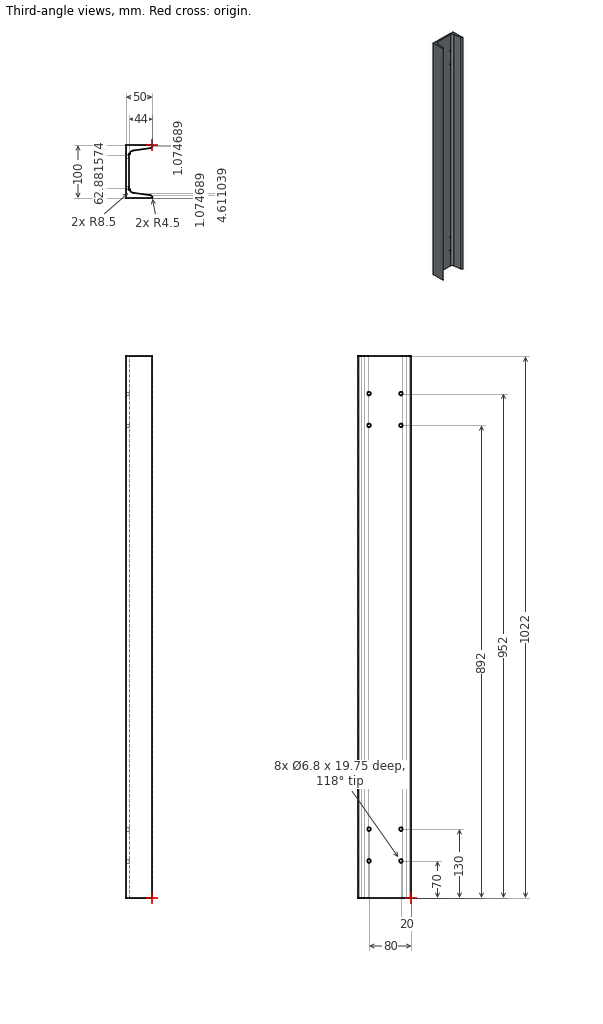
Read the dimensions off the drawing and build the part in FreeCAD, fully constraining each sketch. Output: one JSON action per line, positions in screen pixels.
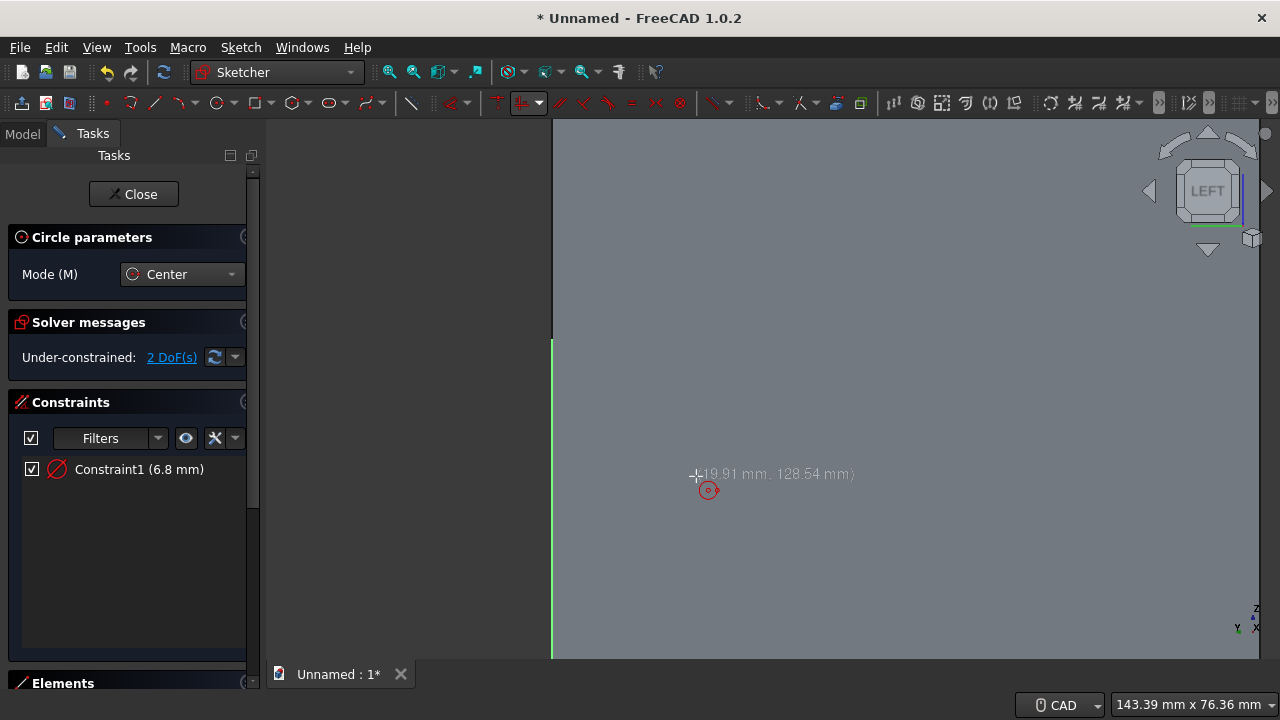
{"action": "scroll", "coordinate": [697, 514], "scroll_direction": "down", "scroll_amount": 15}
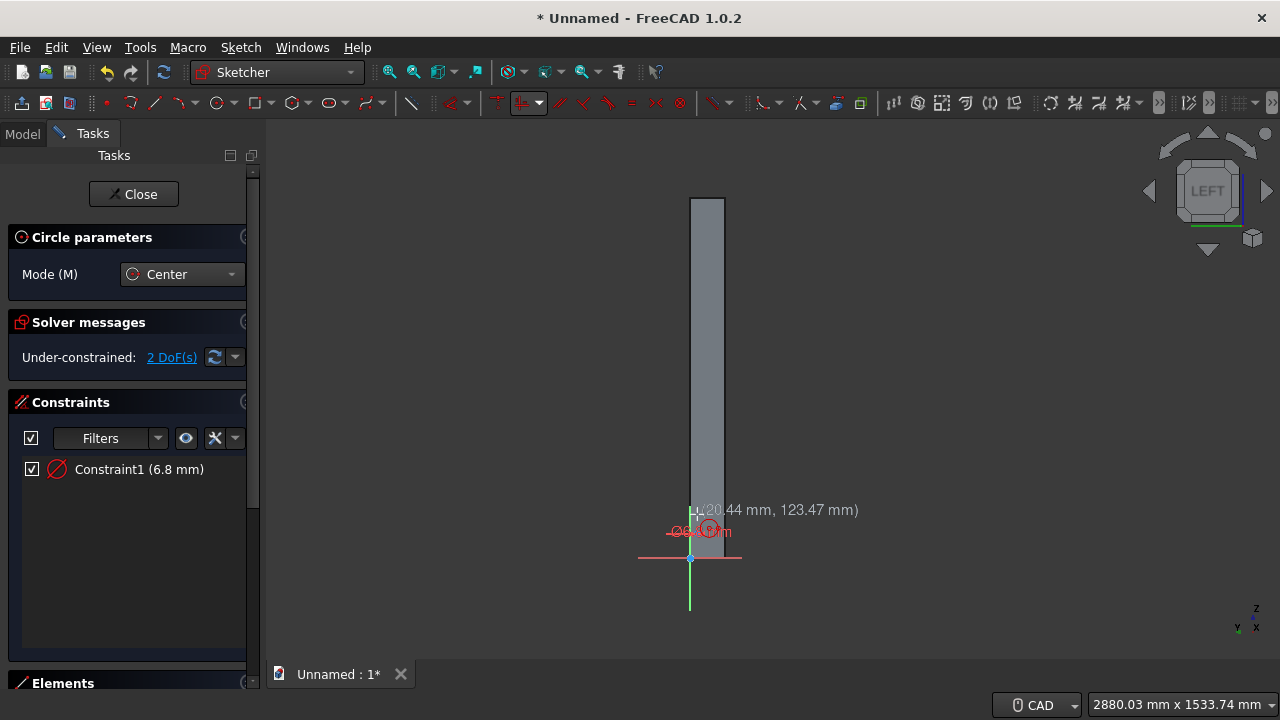
{"action": "scroll", "coordinate": [697, 512], "scroll_direction": "up", "scroll_amount": 5}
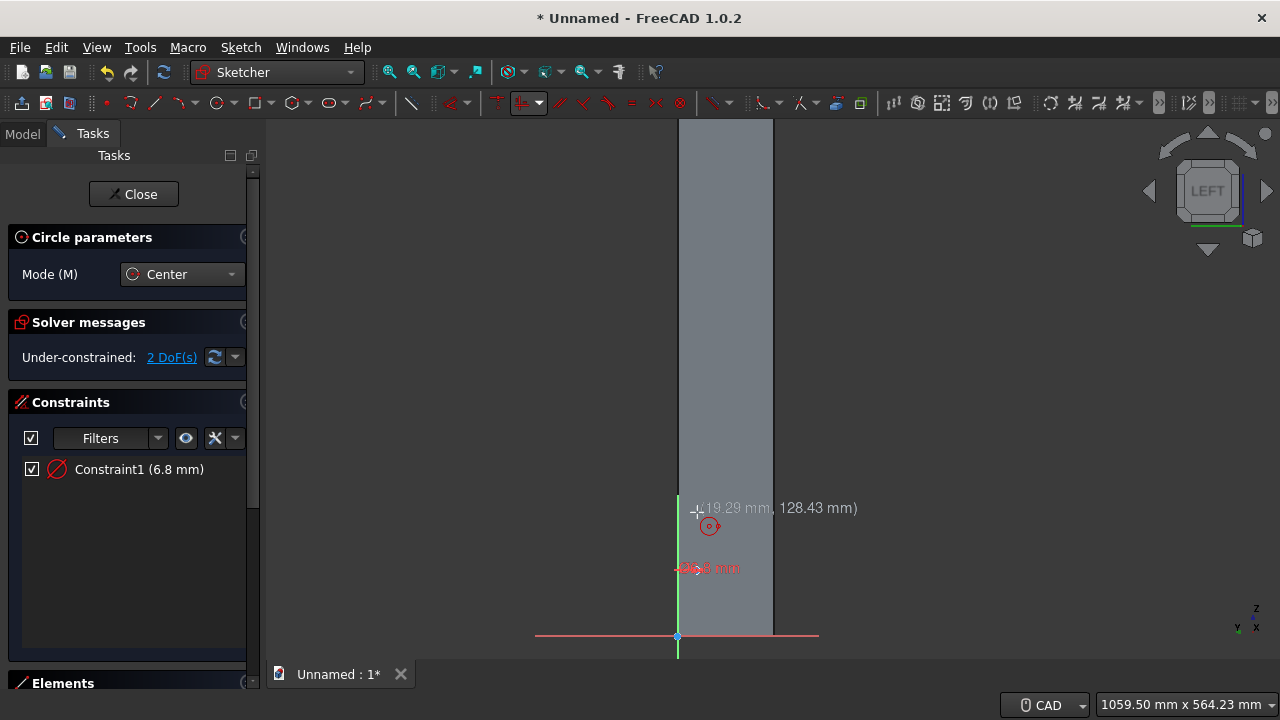
{"action": "left_click", "coordinate": [697, 512]}
{"action": "mouse_move", "coordinate": [699, 510]}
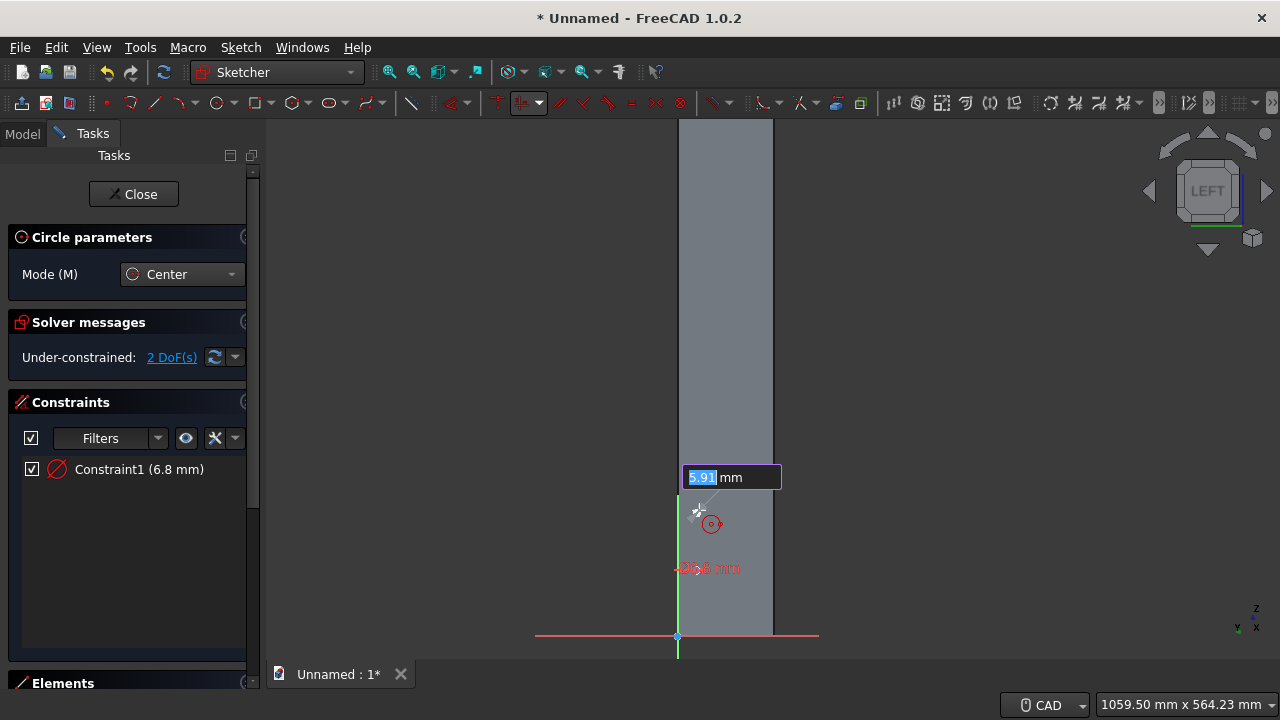
{"action": "type", "text": "6.8"}
{"action": "key", "text": "Return"}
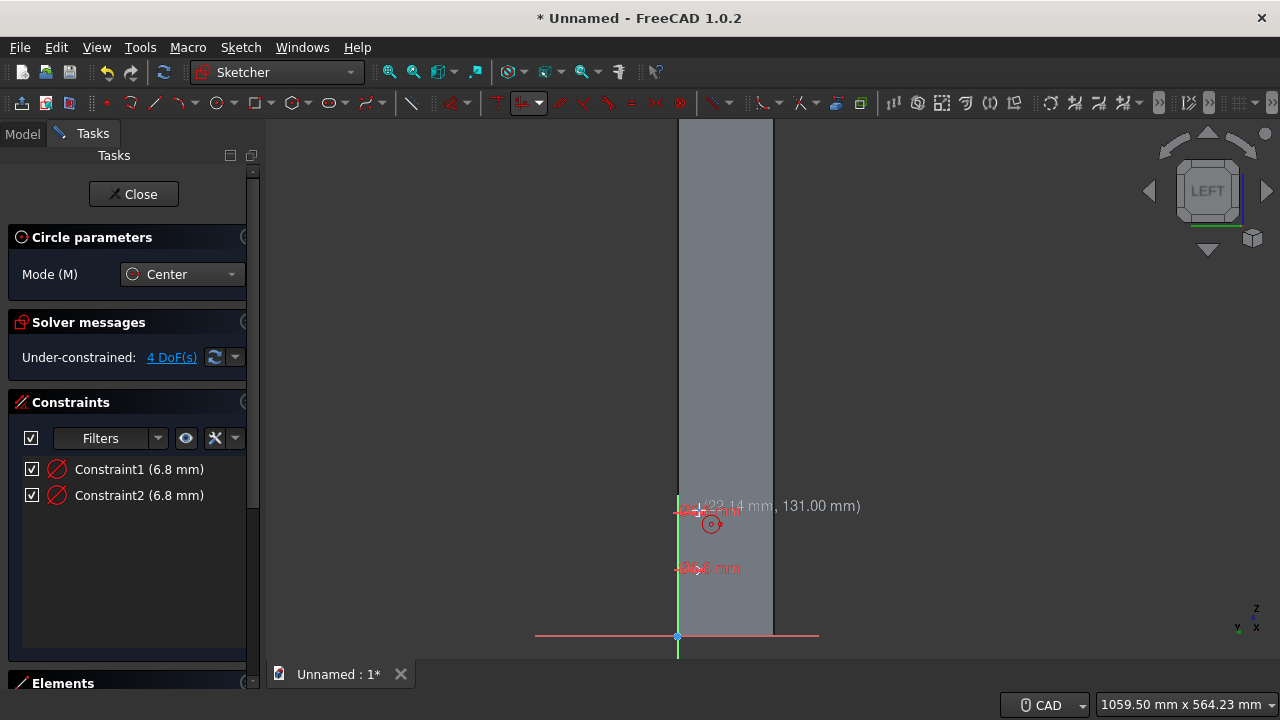
{"action": "scroll", "coordinate": [754, 512], "scroll_direction": "up", "scroll_amount": 10}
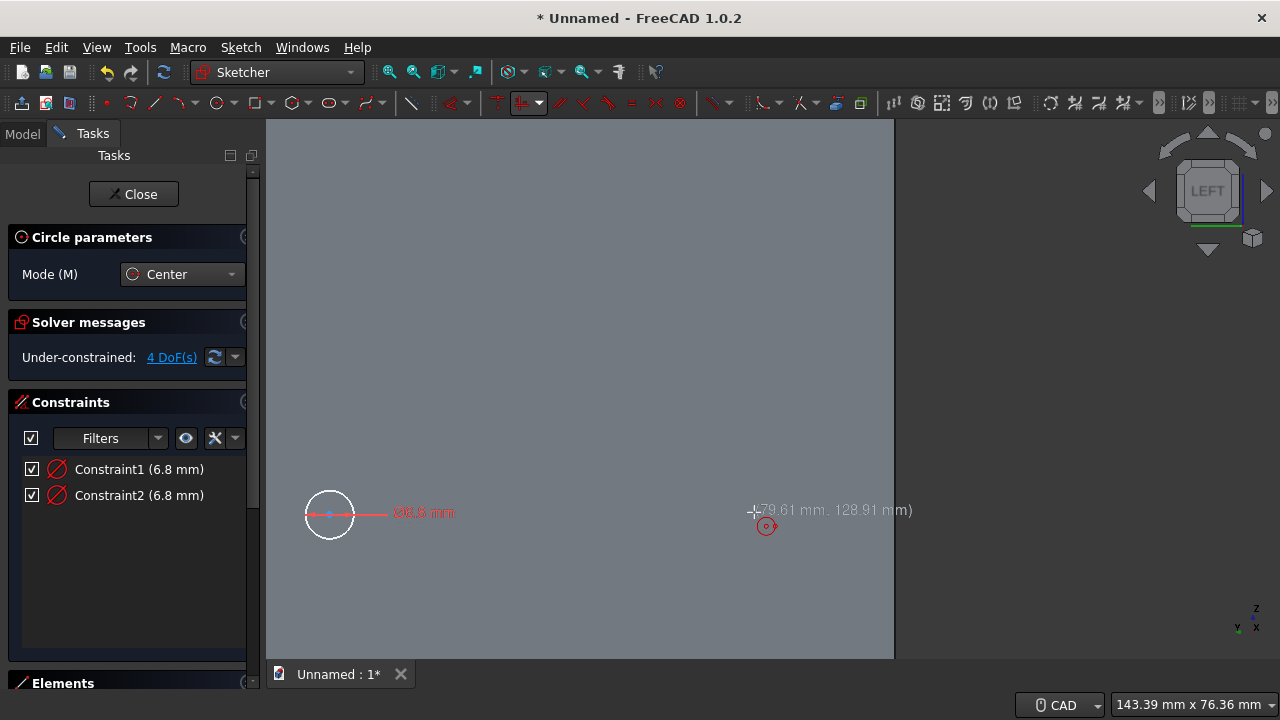
{"action": "scroll", "coordinate": [716, 512], "scroll_direction": "down", "scroll_amount": 15}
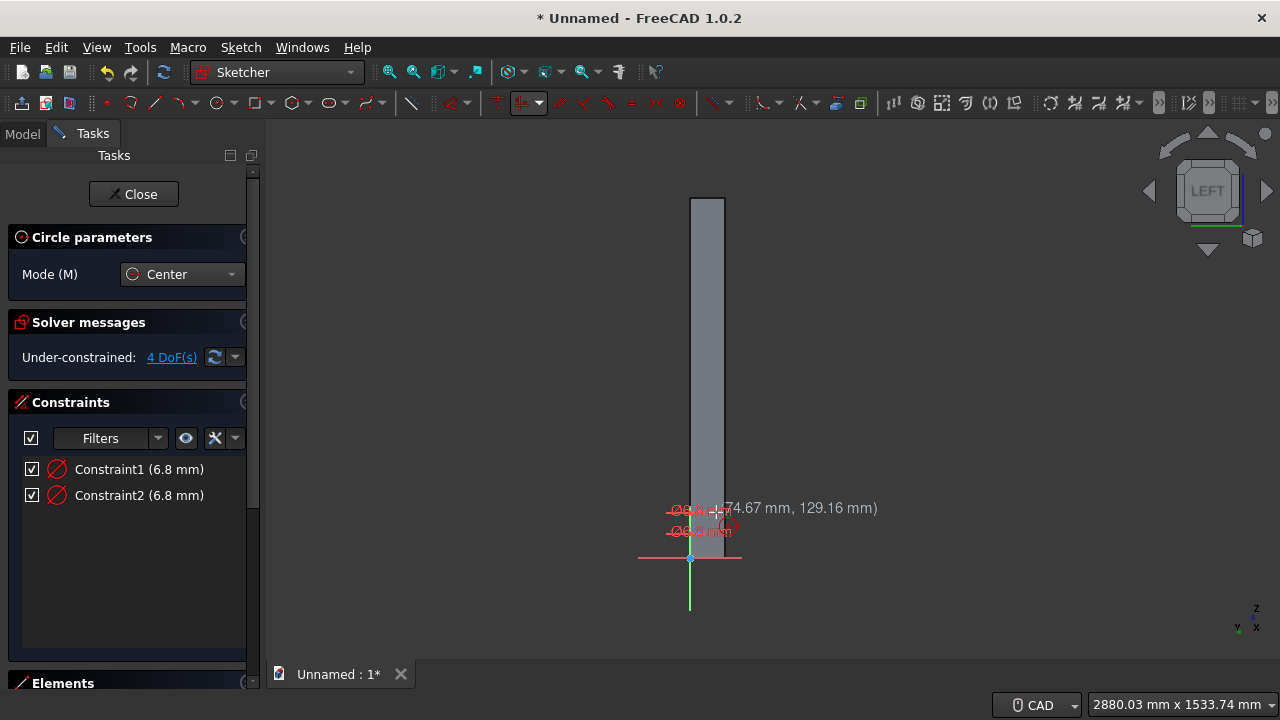
{"action": "left_click", "coordinate": [718, 512]}
{"action": "mouse_move", "coordinate": [719, 512]}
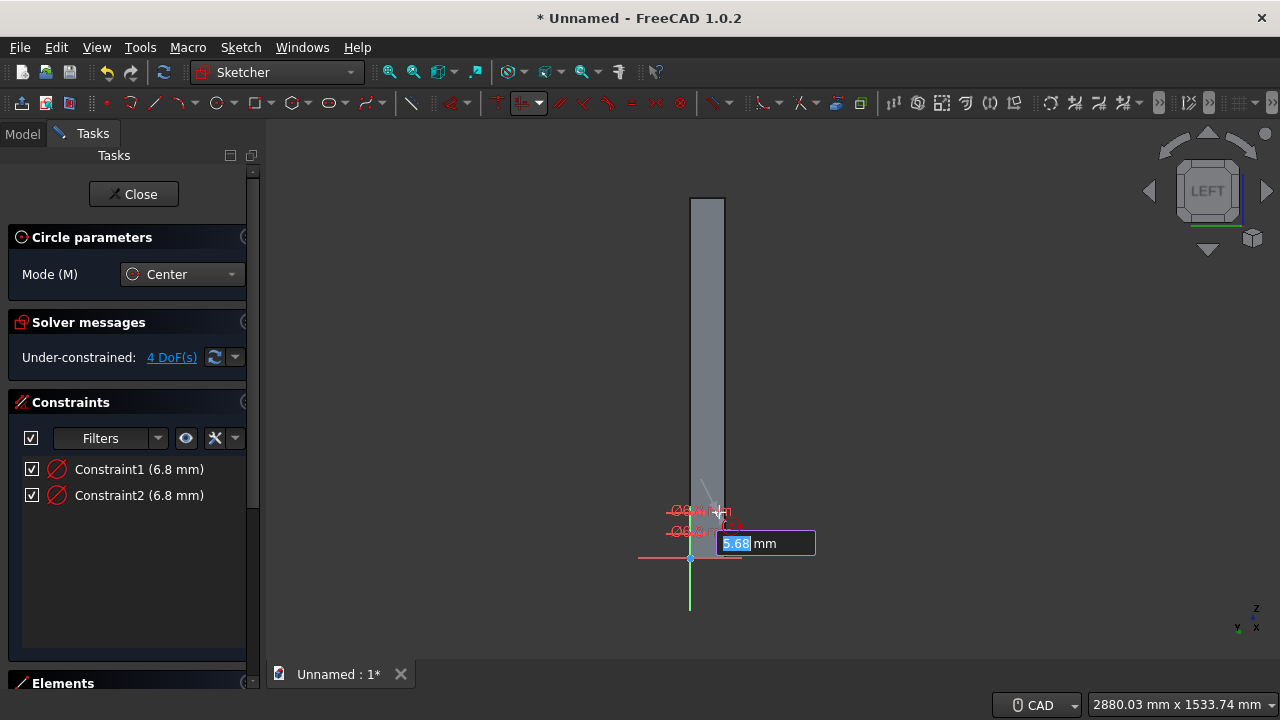
{"action": "type", "text": "6.8"}
{"action": "key", "text": "Return"}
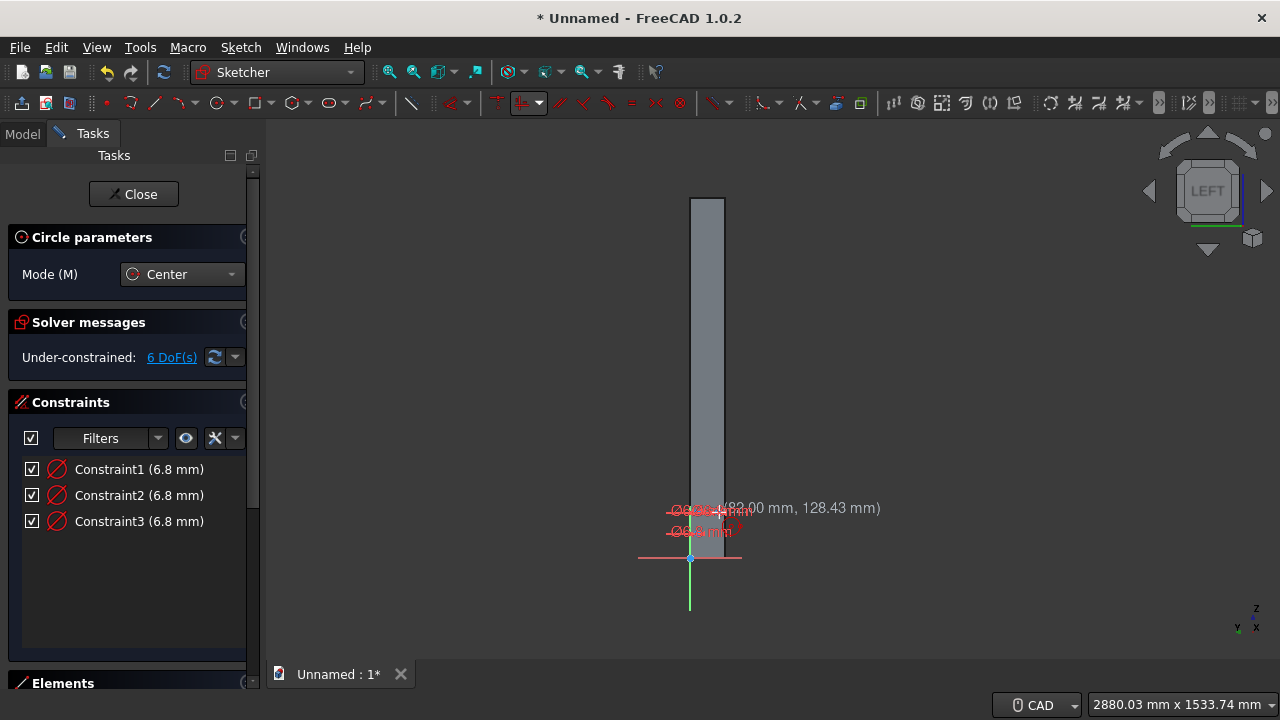
{"action": "scroll", "coordinate": [718, 534], "scroll_direction": "up", "scroll_amount": 15}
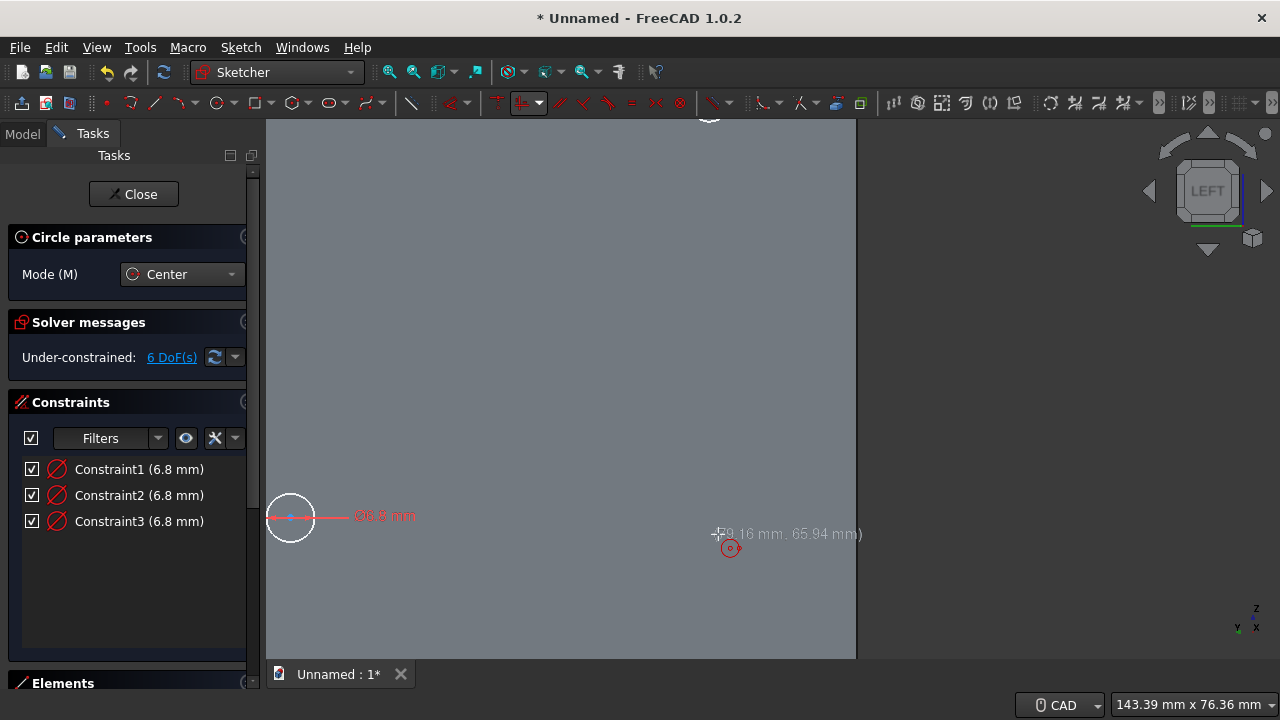
{"action": "scroll", "coordinate": [718, 534], "scroll_direction": "down", "scroll_amount": 15}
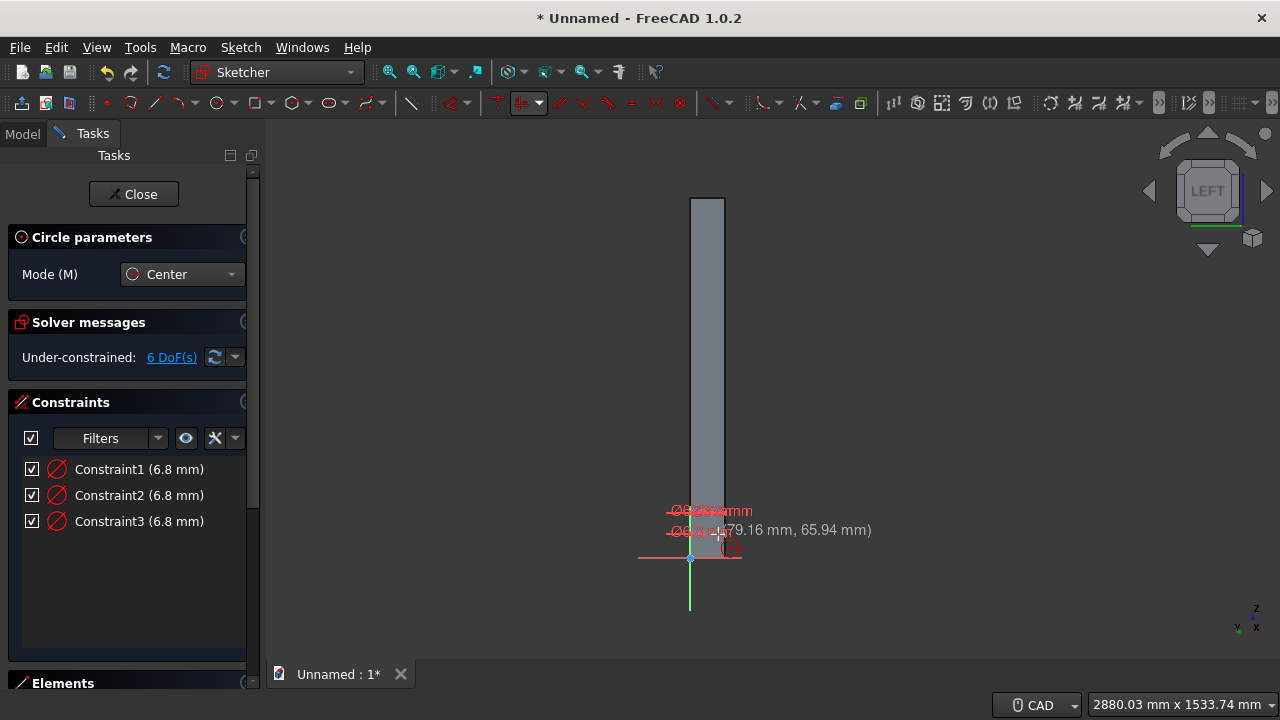
{"action": "left_click", "coordinate": [718, 534]}
{"action": "mouse_move", "coordinate": [719, 533]}